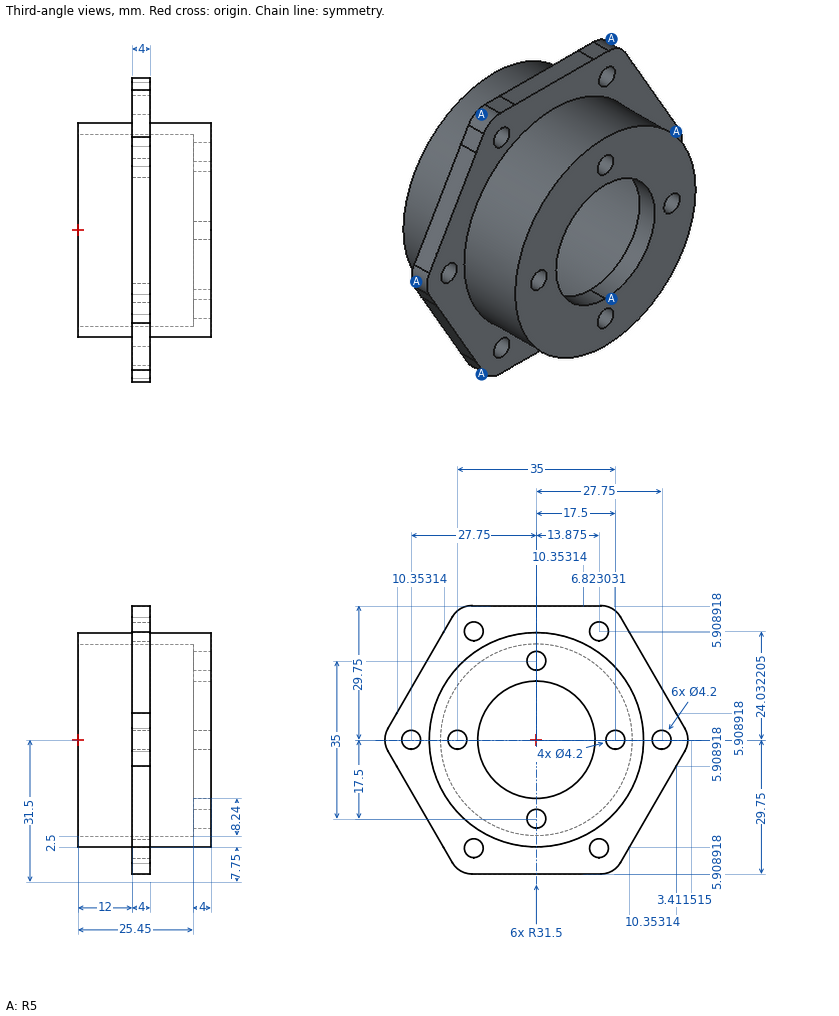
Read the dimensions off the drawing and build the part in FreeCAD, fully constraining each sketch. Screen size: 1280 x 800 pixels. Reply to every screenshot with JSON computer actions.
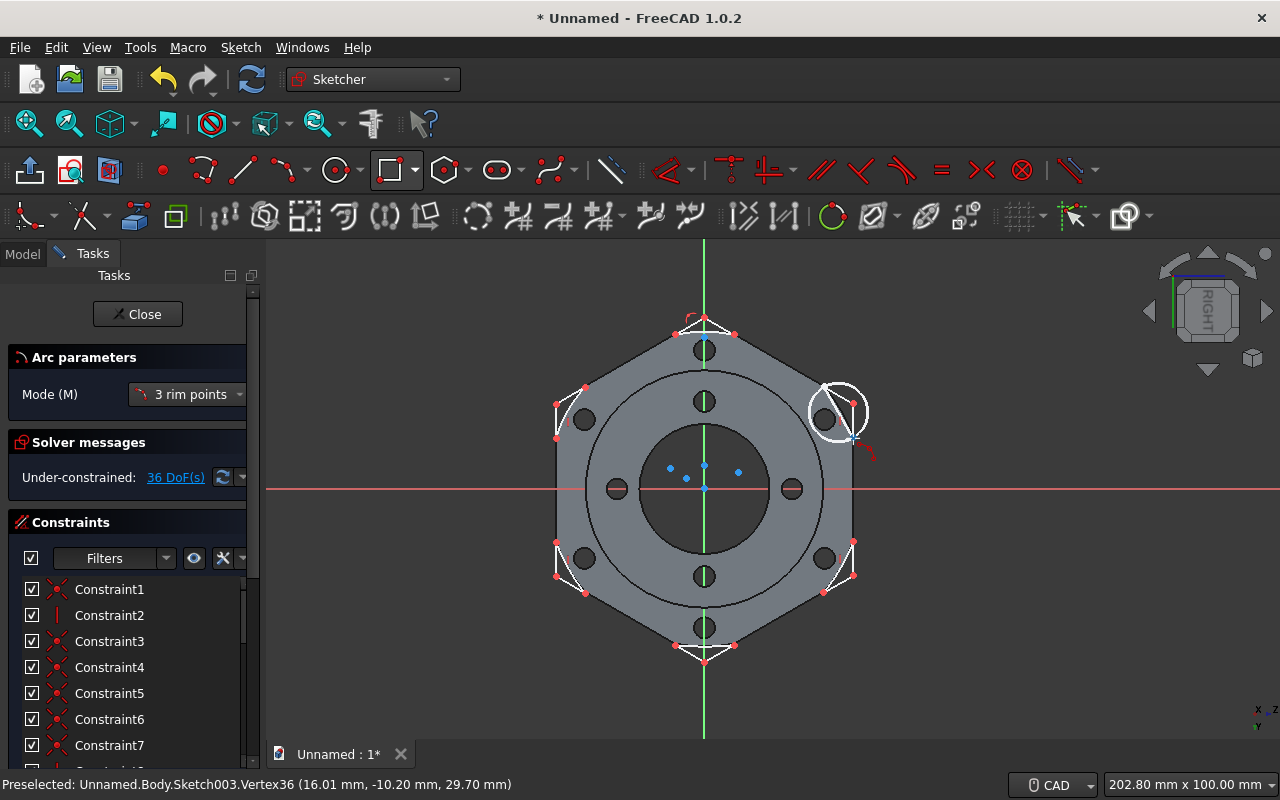
{"action": "scroll", "coordinate": [841, 410], "scroll_direction": "up", "scroll_amount": 9}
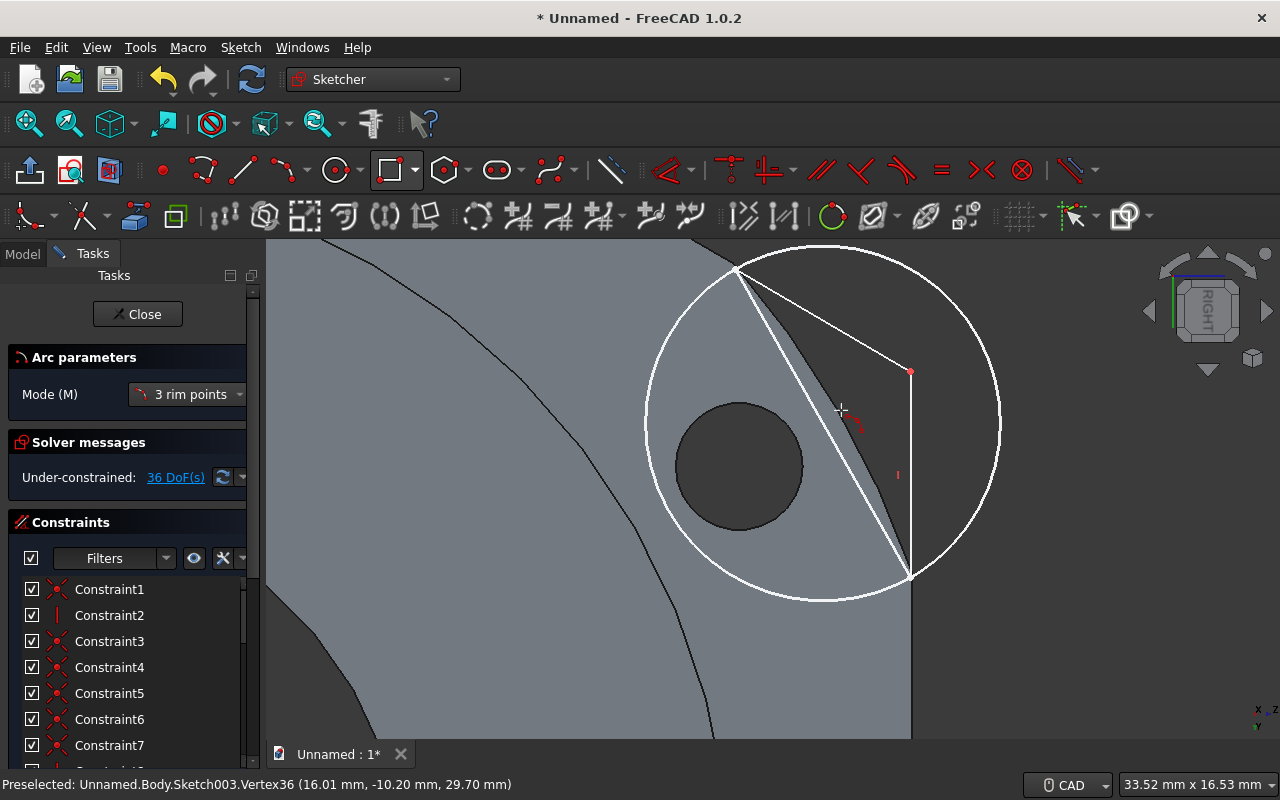
{"action": "left_click", "coordinate": [837, 410]}
{"action": "key", "text": "Escape"}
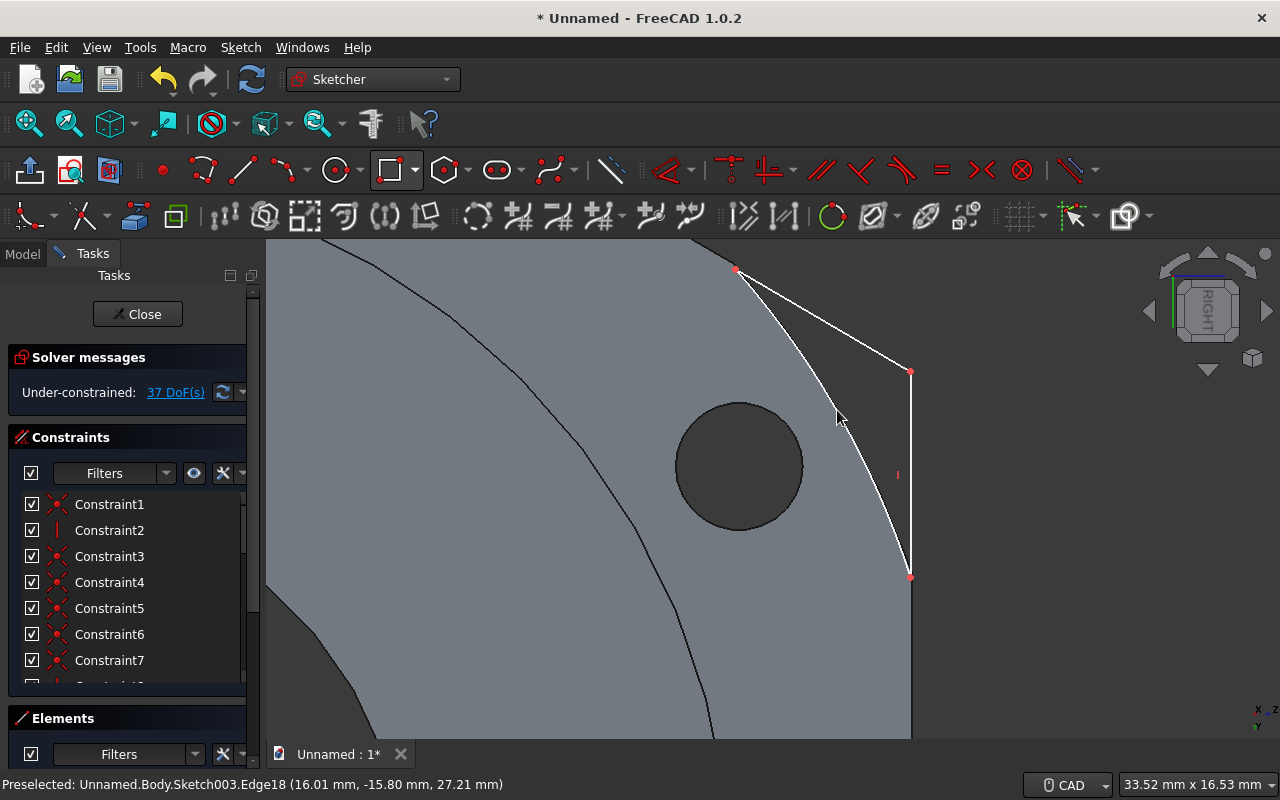
{"action": "scroll", "coordinate": [842, 410], "scroll_direction": "down", "scroll_amount": 9}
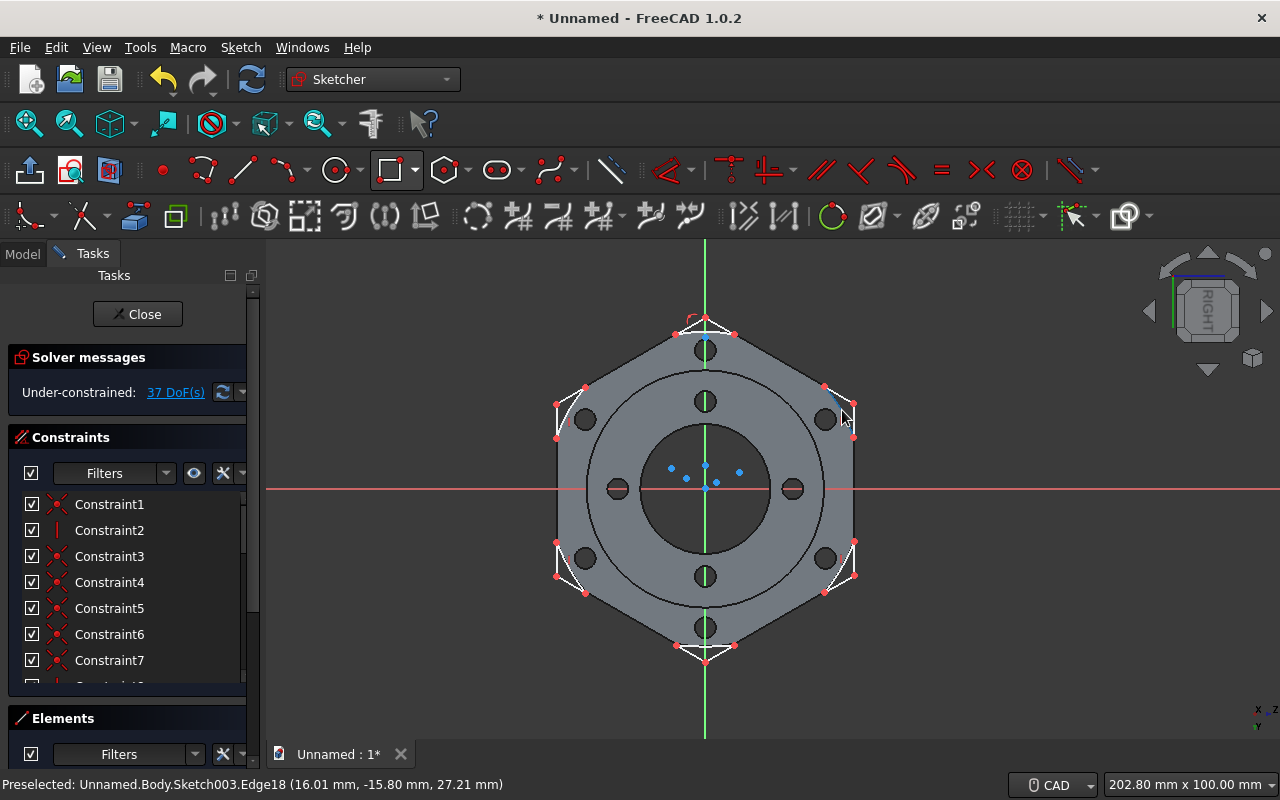
{"action": "scroll", "coordinate": [835, 579], "scroll_direction": "up", "scroll_amount": 4}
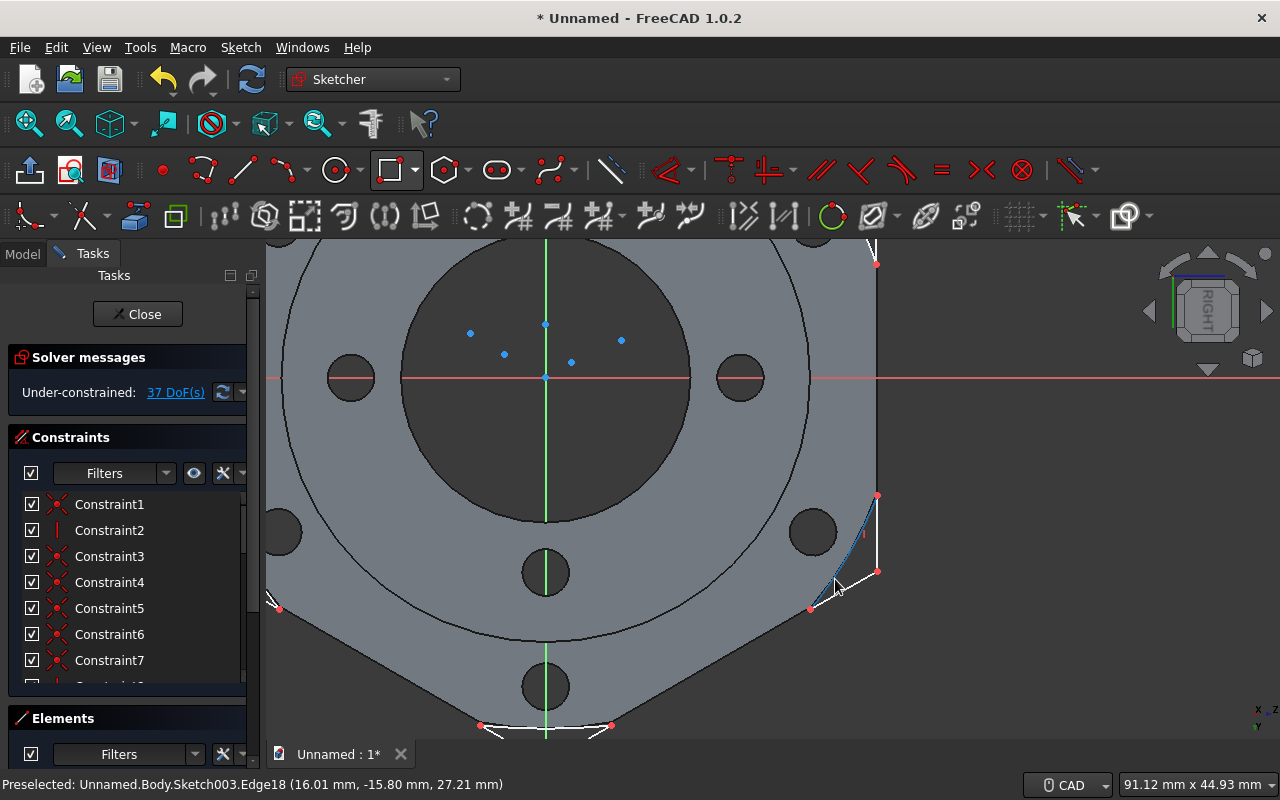
{"action": "left_click", "coordinate": [834, 577]}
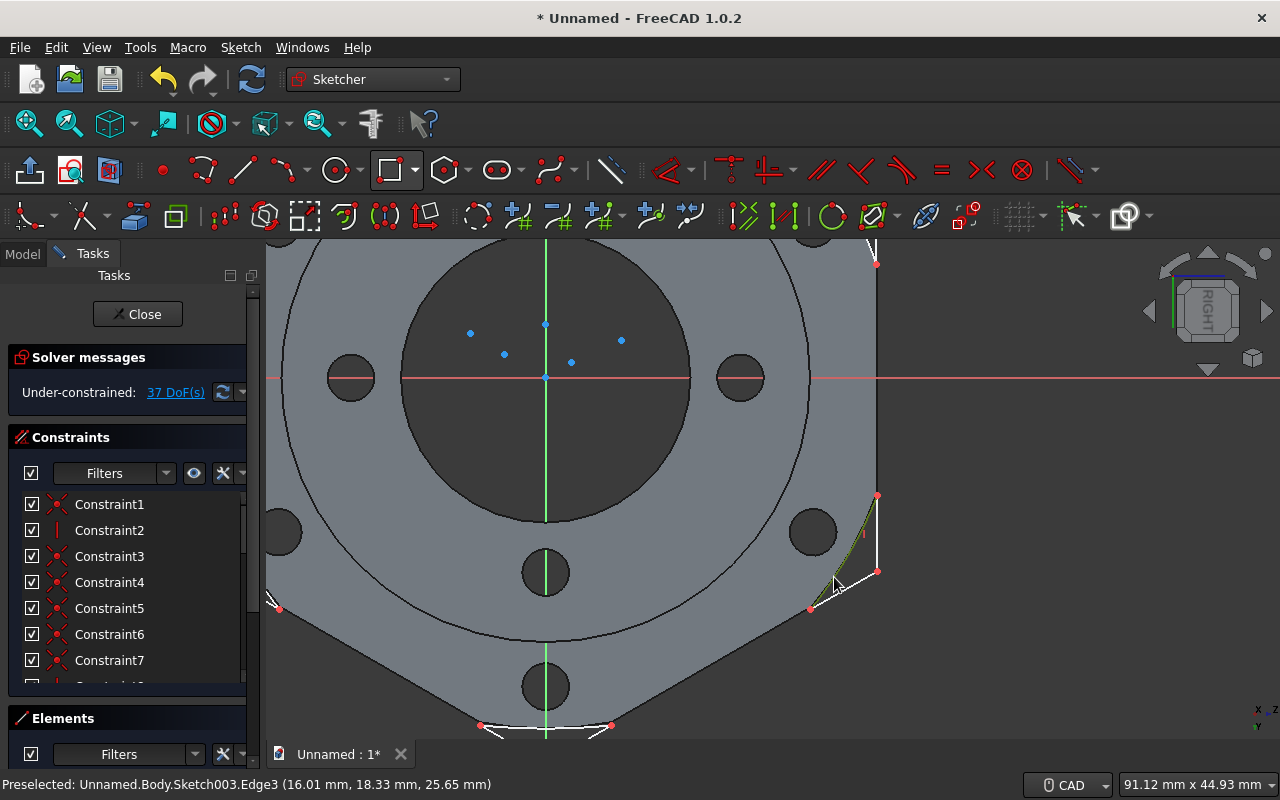
{"action": "scroll", "coordinate": [834, 580], "scroll_direction": "down", "scroll_amount": 4}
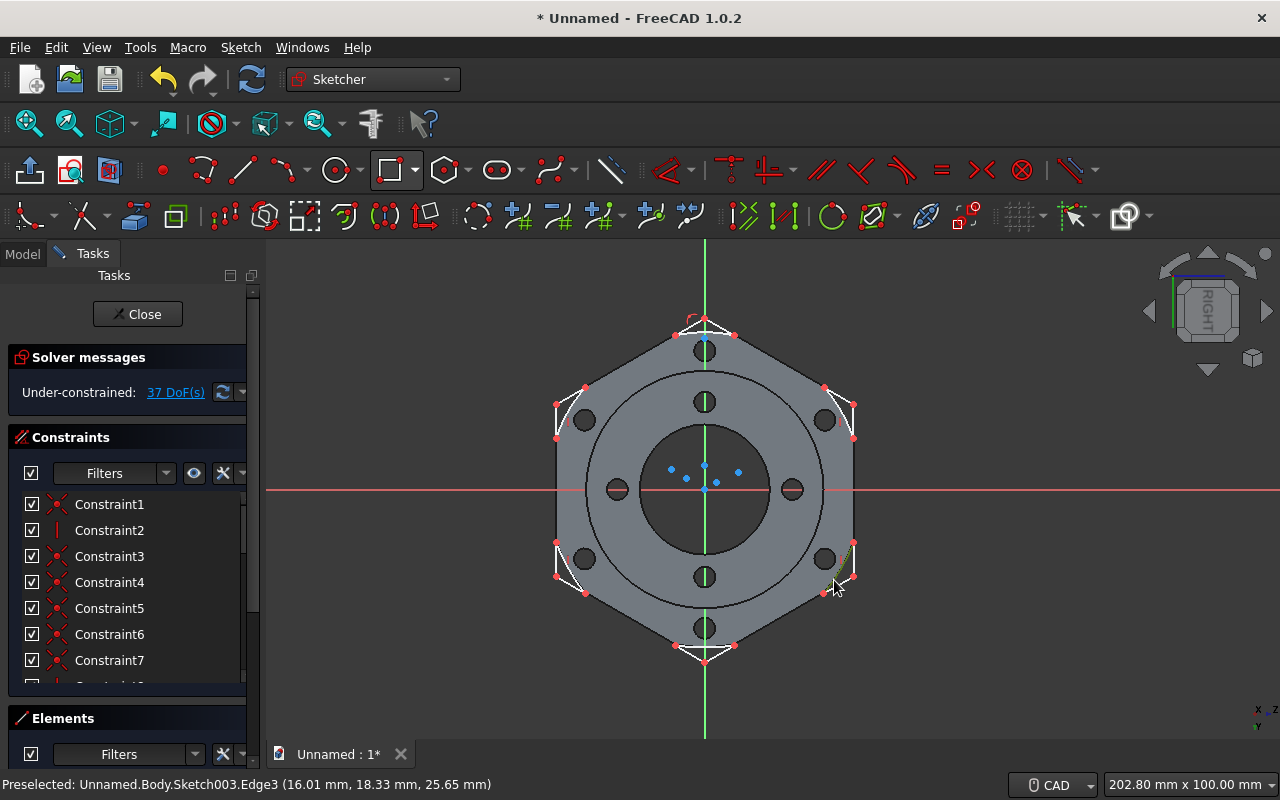
{"action": "scroll", "coordinate": [693, 647], "scroll_direction": "up", "scroll_amount": 3}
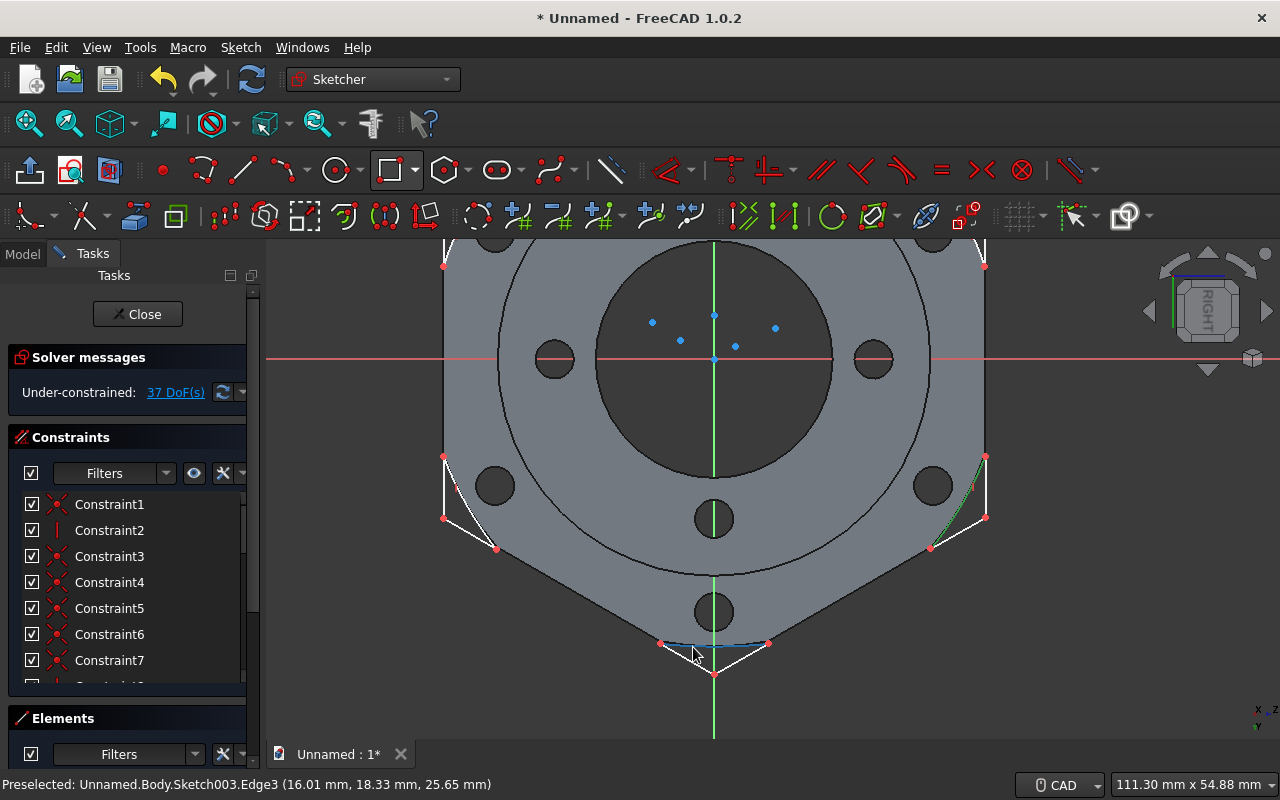
{"action": "left_click", "coordinate": [693, 646]}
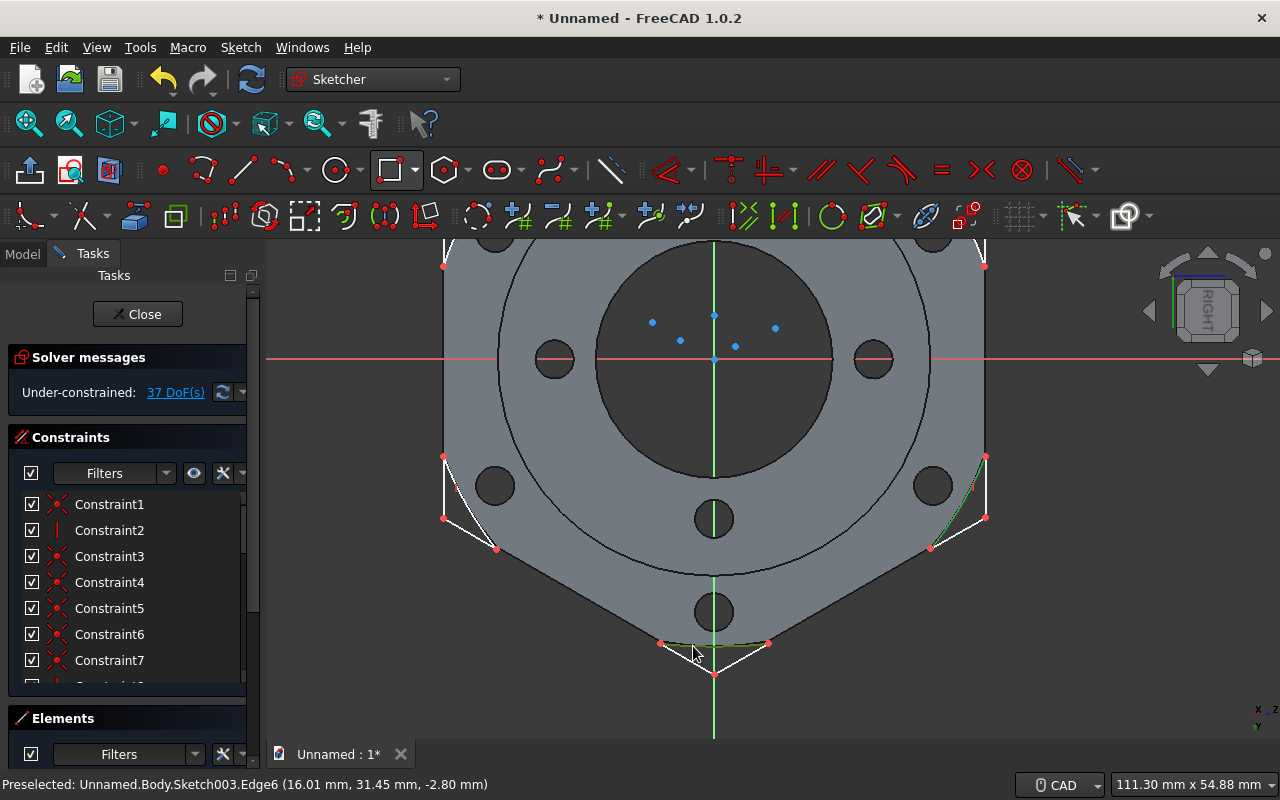
{"action": "left_click", "coordinate": [730, 170]}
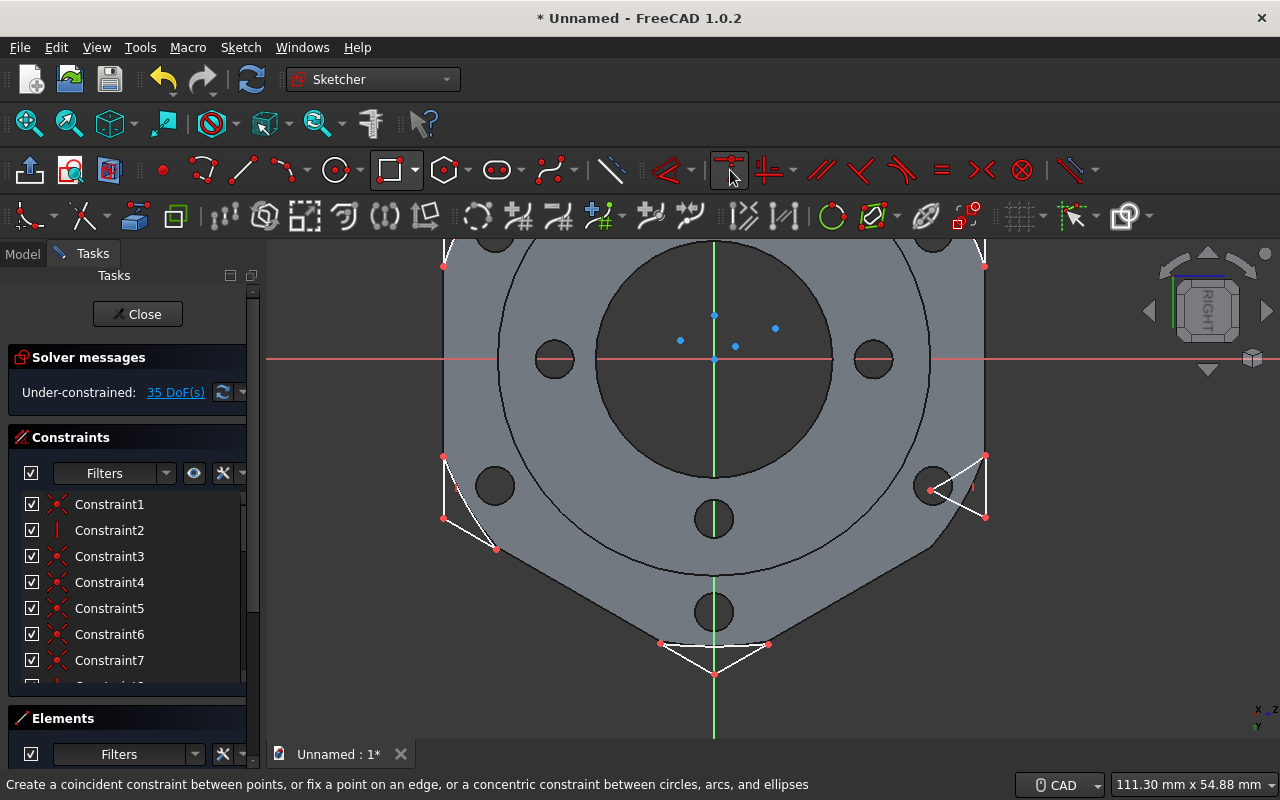
{"action": "left_click", "coordinate": [948, 481]}